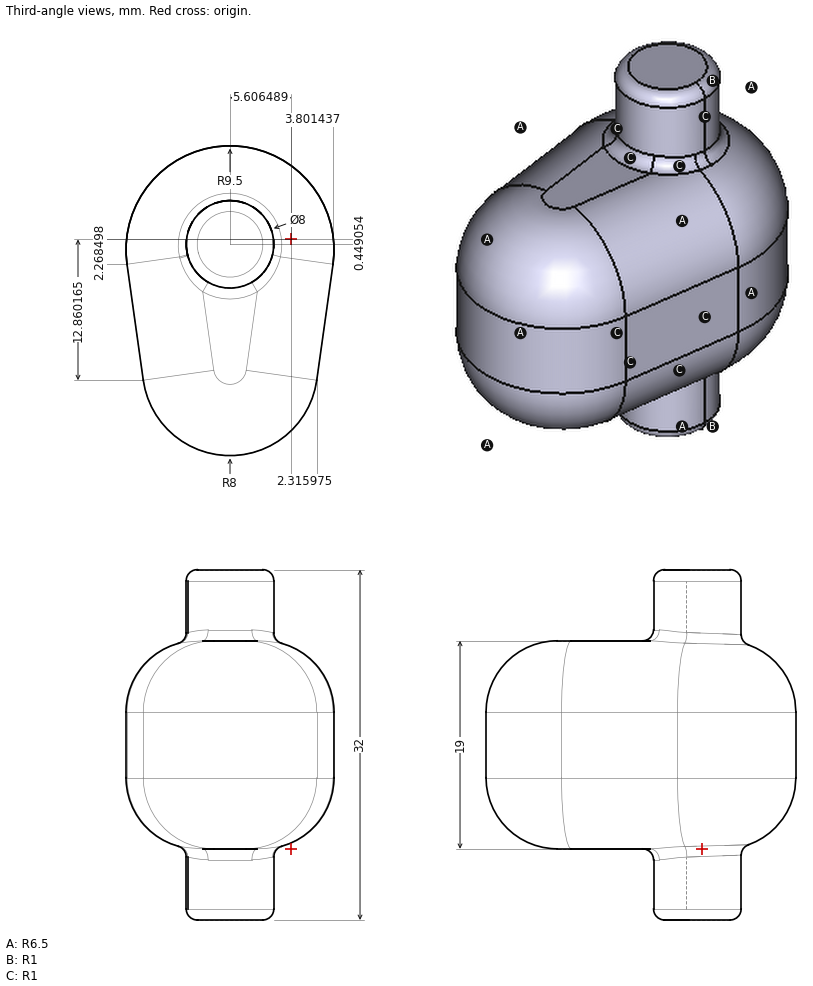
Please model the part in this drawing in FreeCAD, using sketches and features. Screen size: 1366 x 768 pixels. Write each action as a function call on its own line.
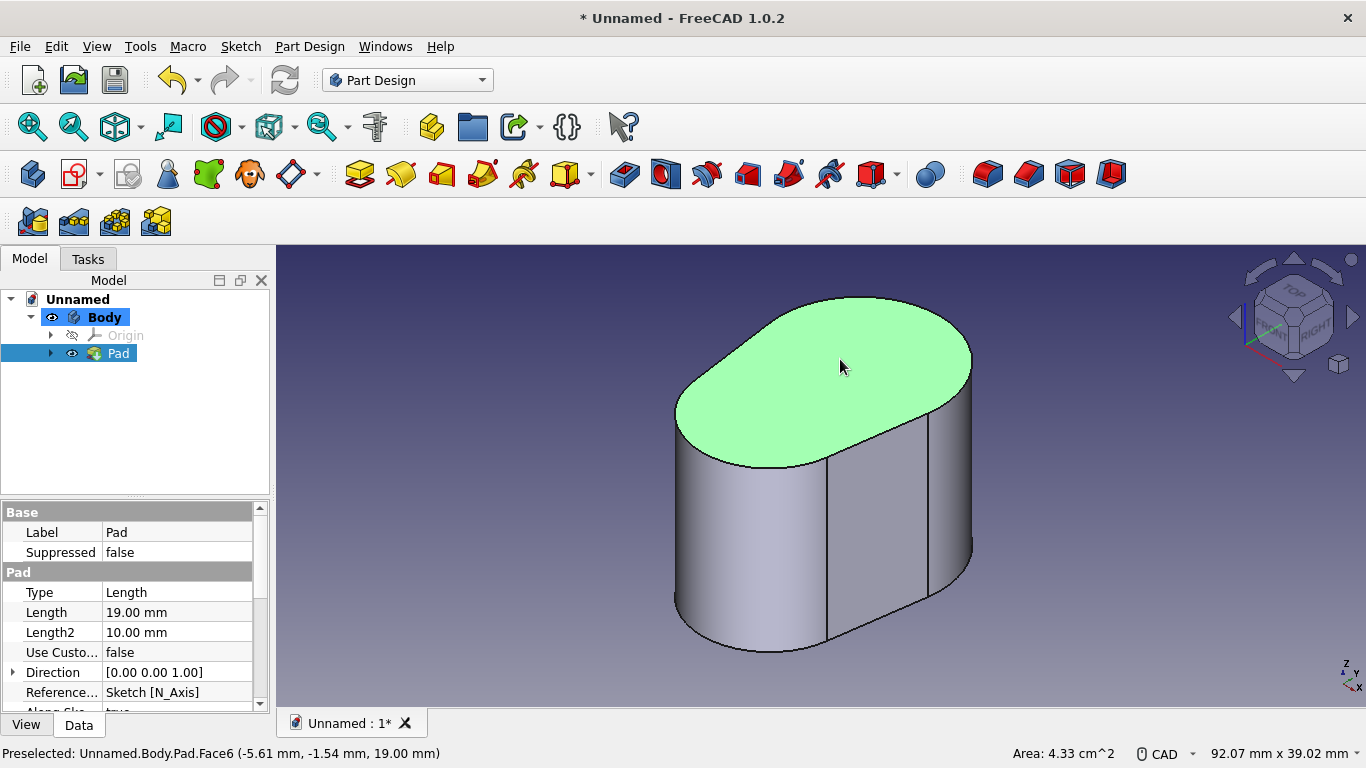
key(2)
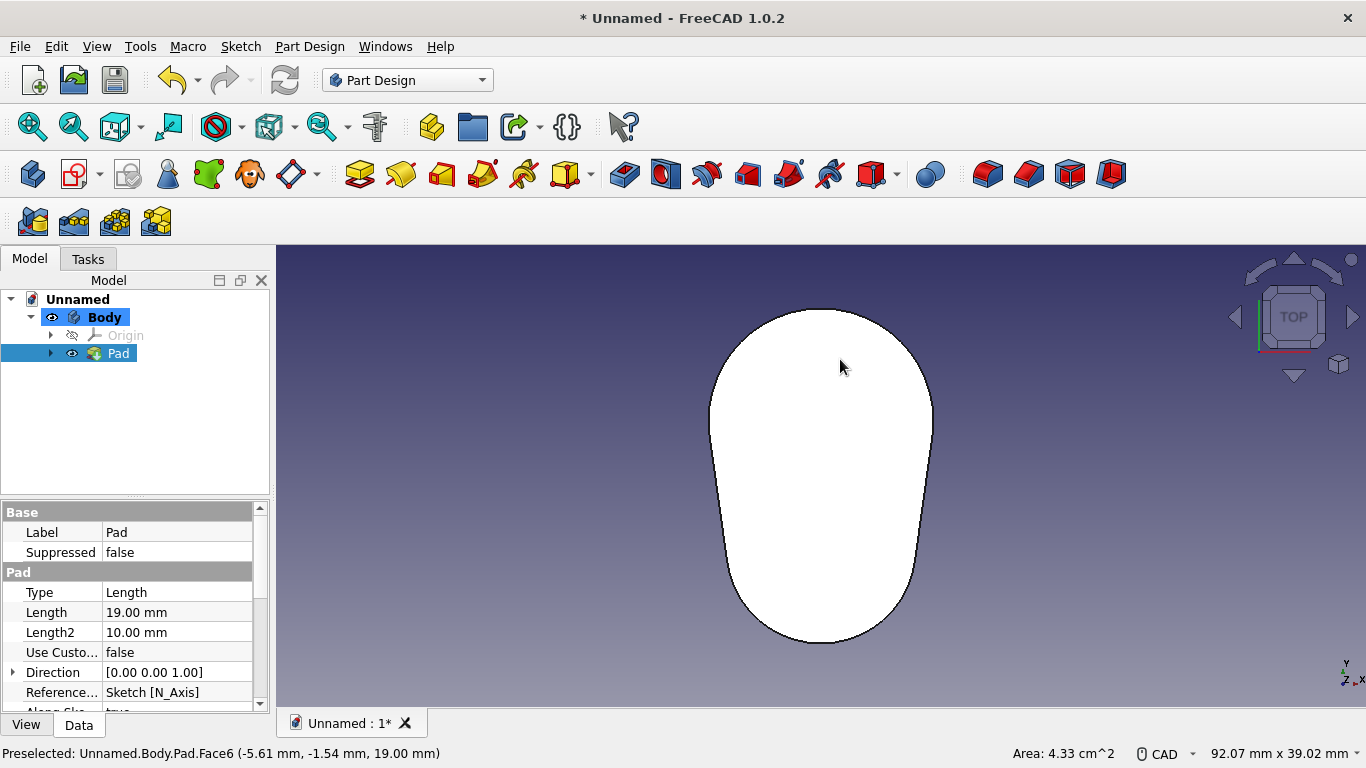
key(1)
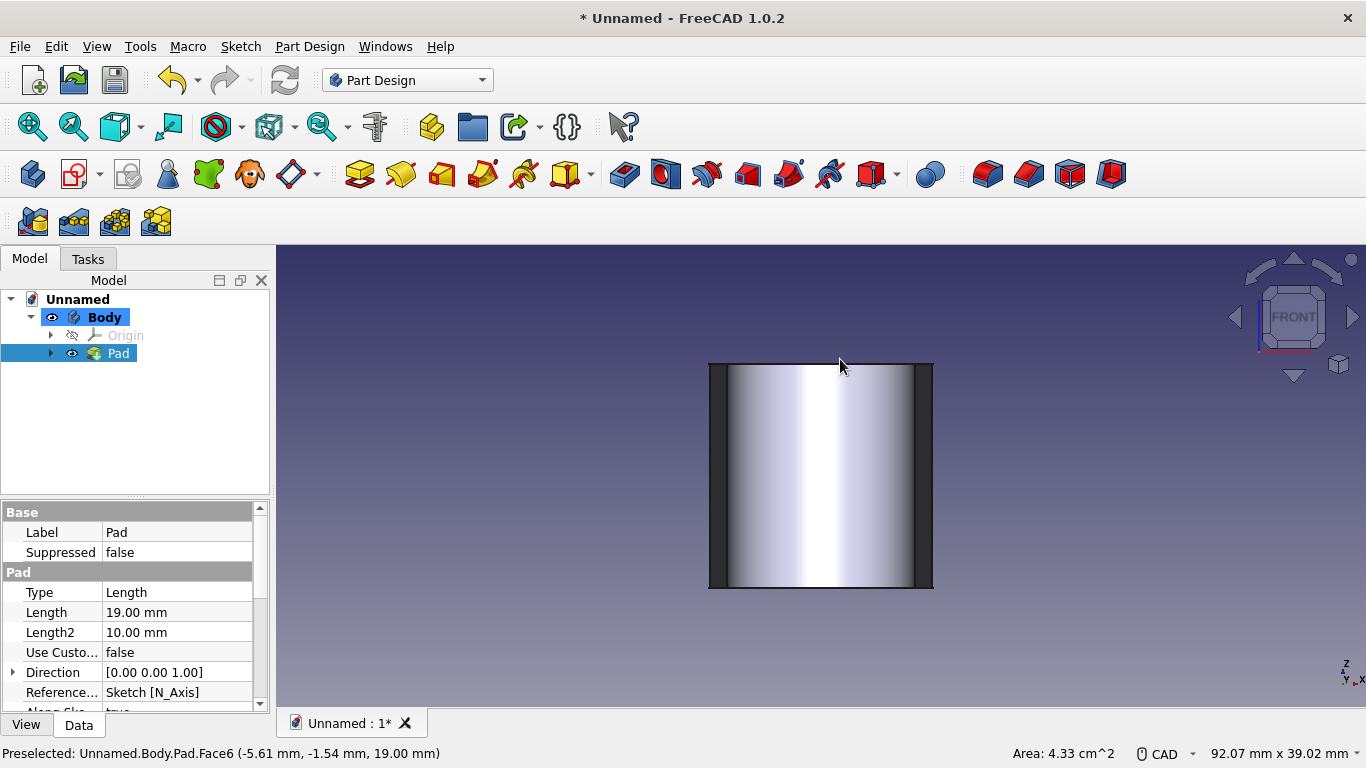
key(3)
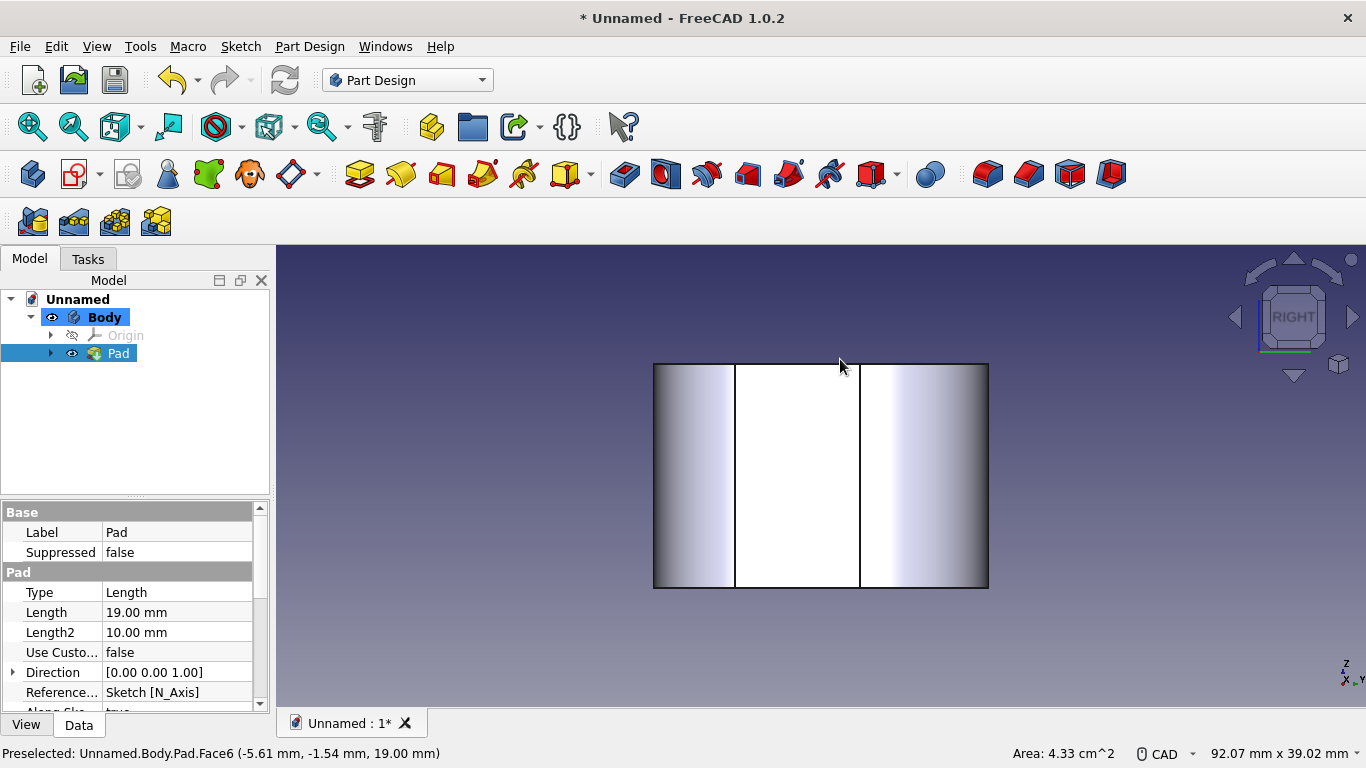
key(5)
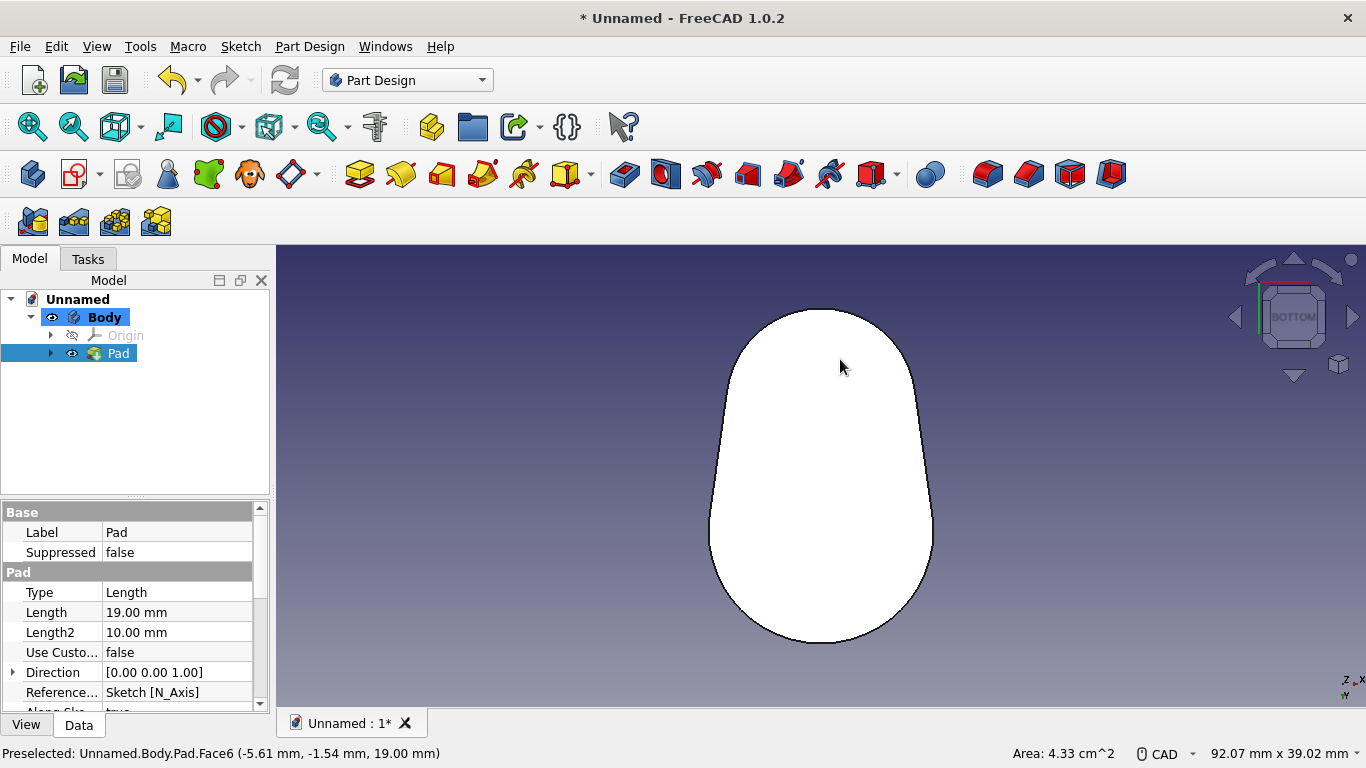
click(821, 523, ctrl)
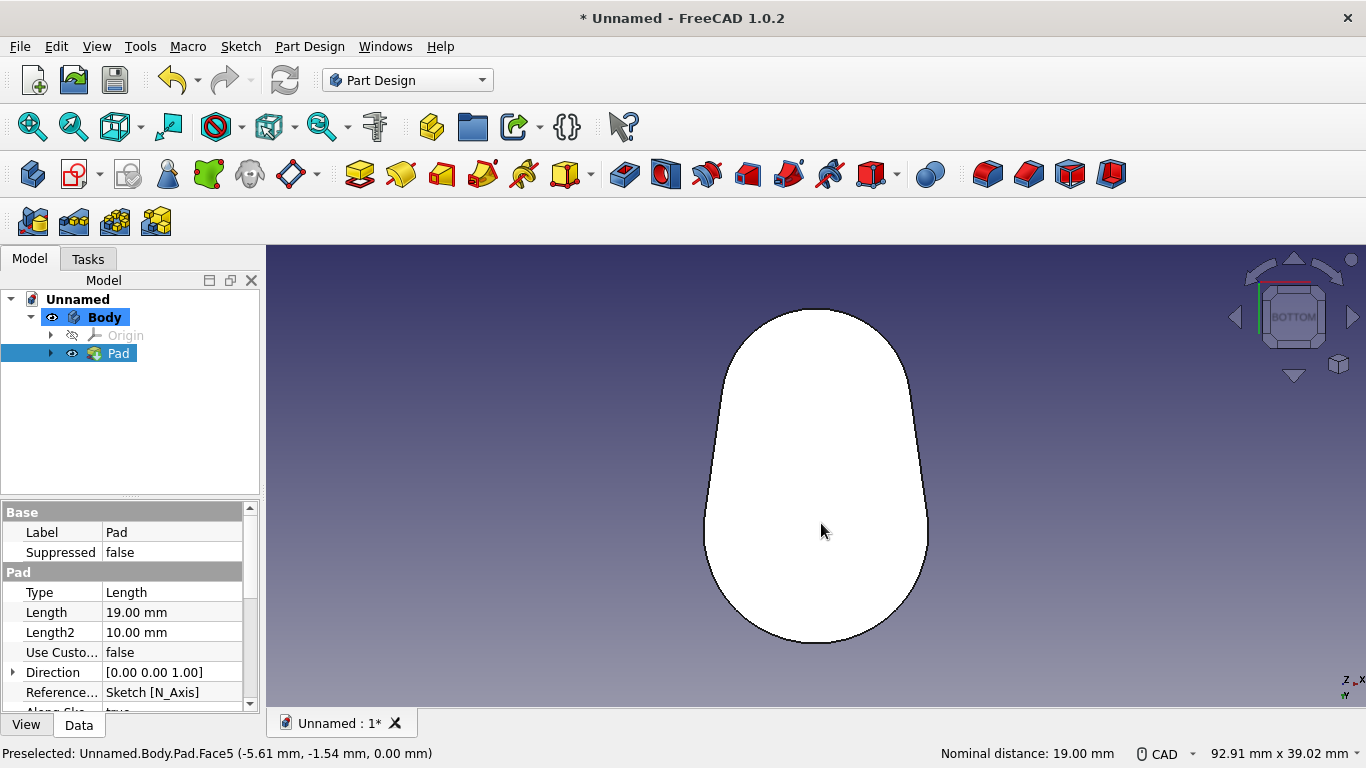
click(988, 174)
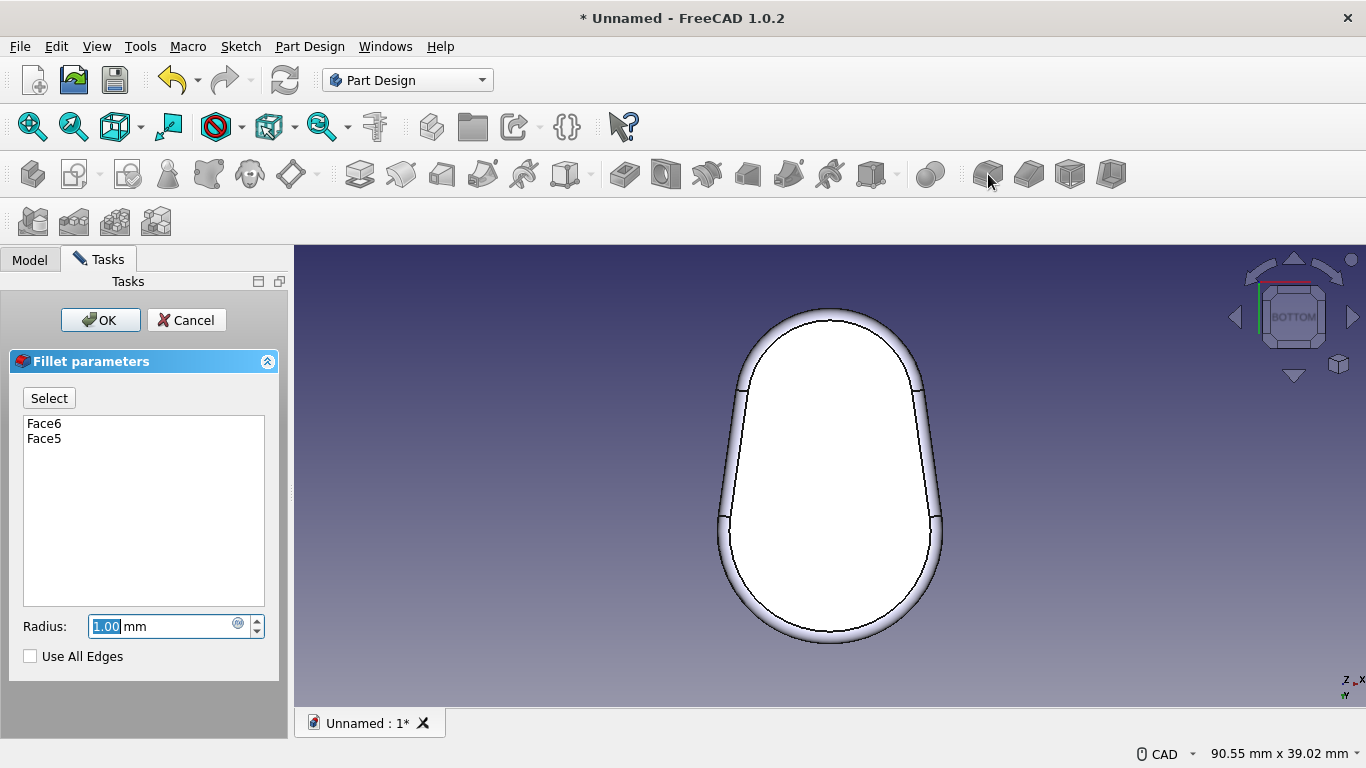
text(6.5)
key(Tab)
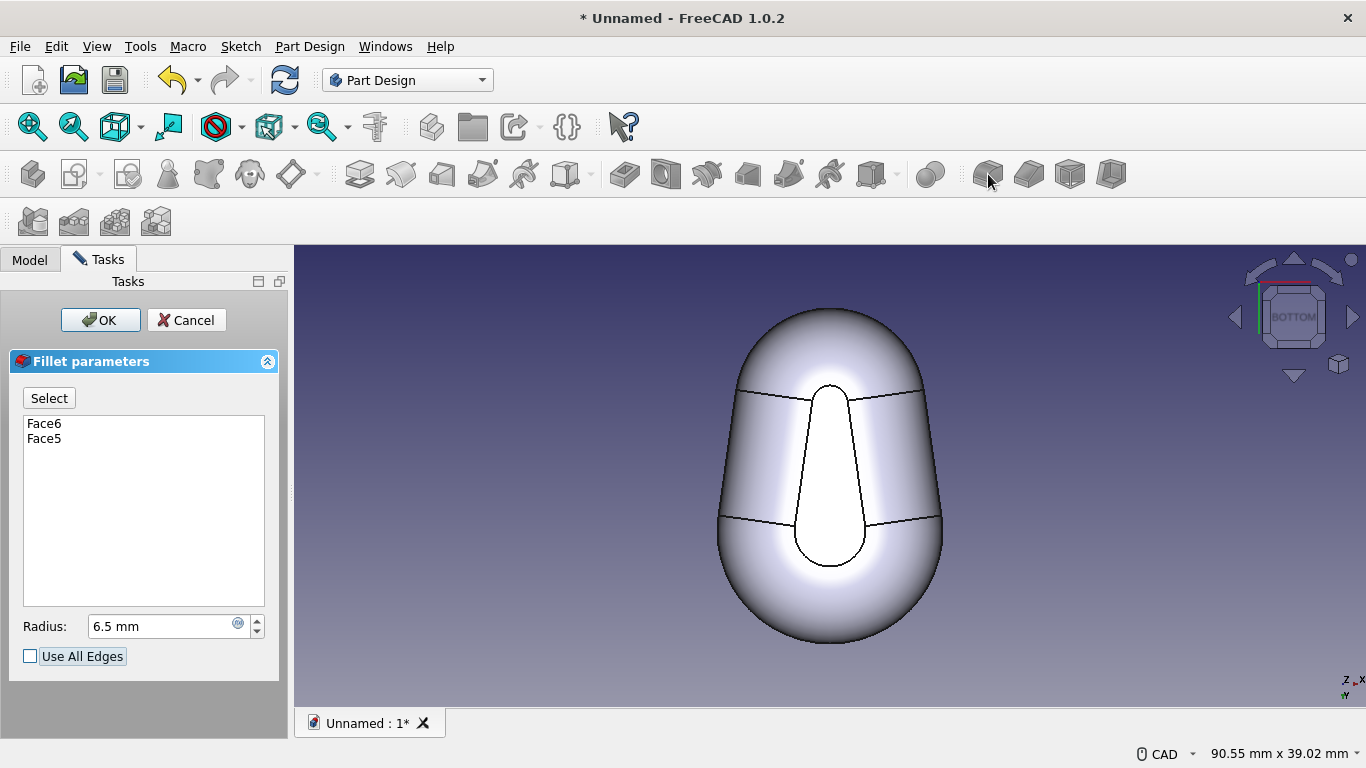
click(101, 320)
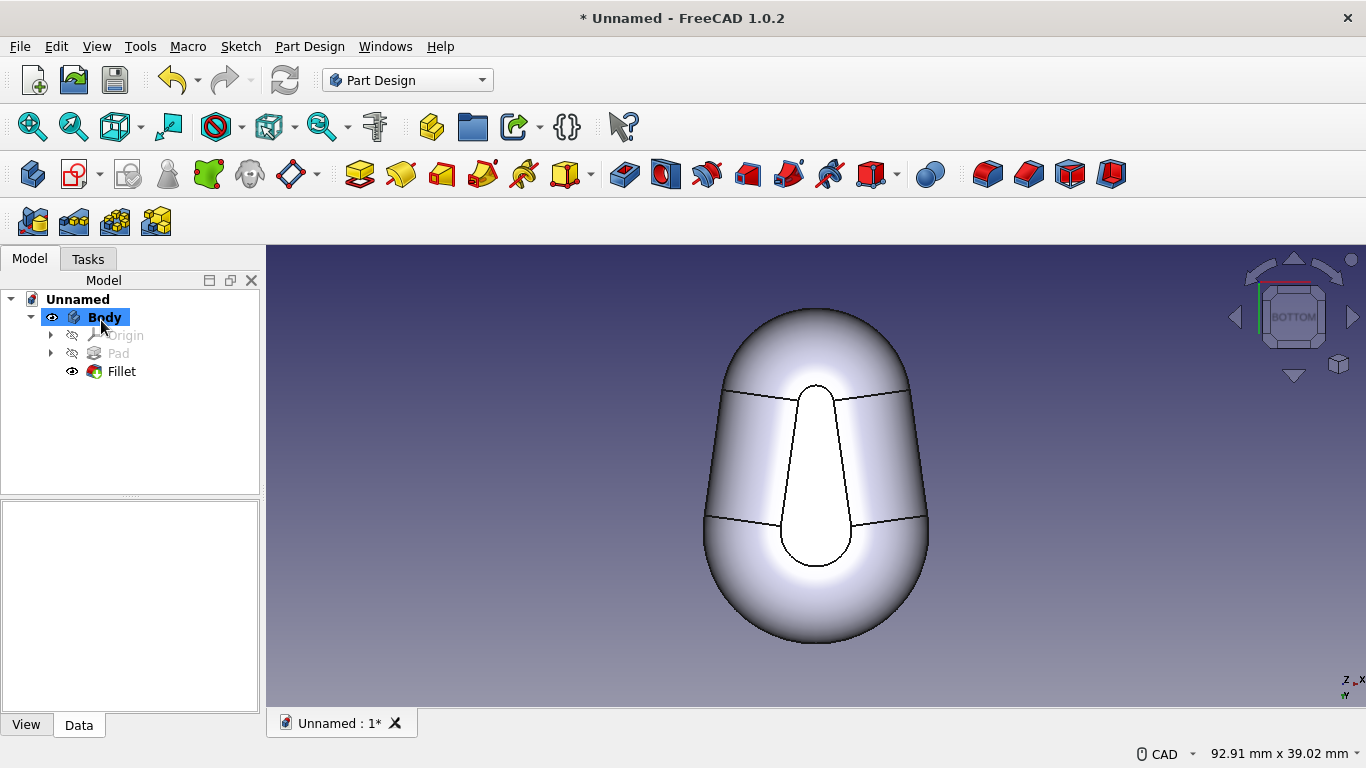
click(51, 335)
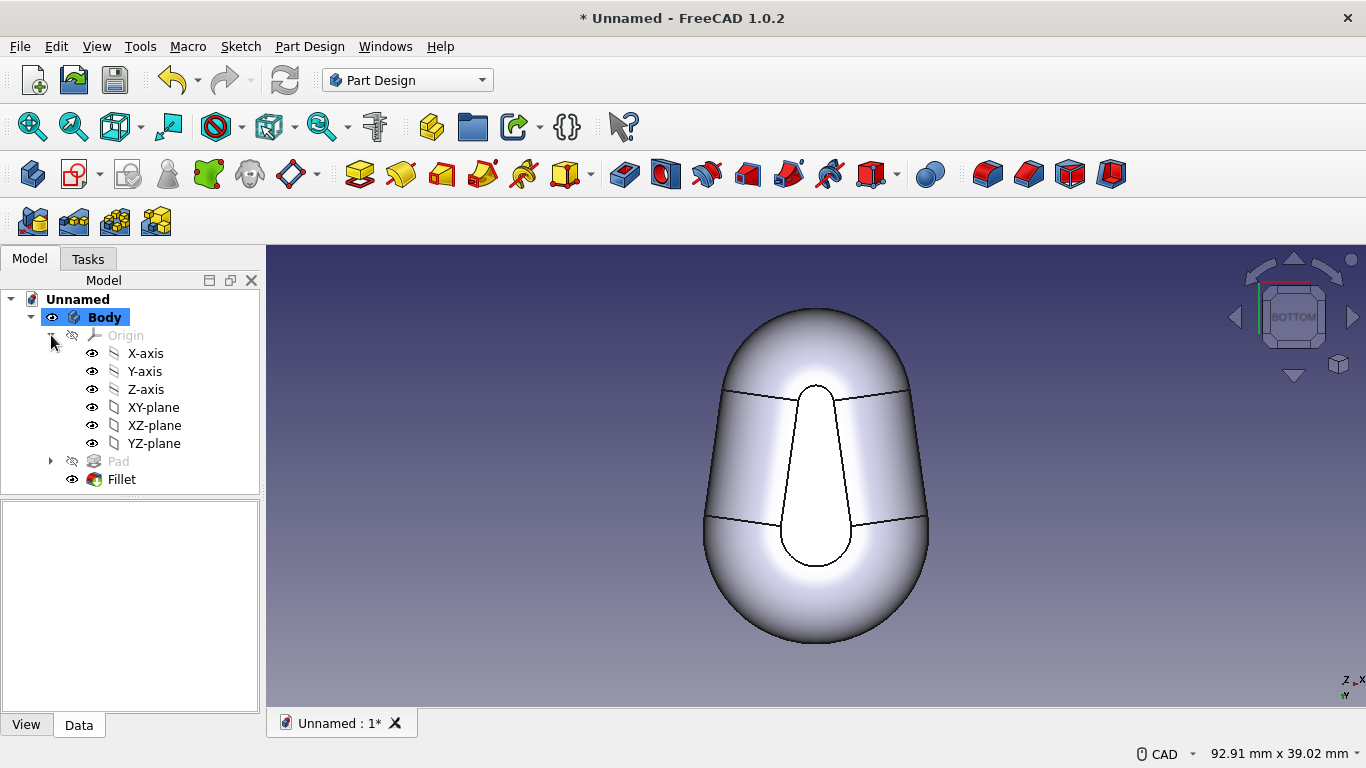
click(137, 407)